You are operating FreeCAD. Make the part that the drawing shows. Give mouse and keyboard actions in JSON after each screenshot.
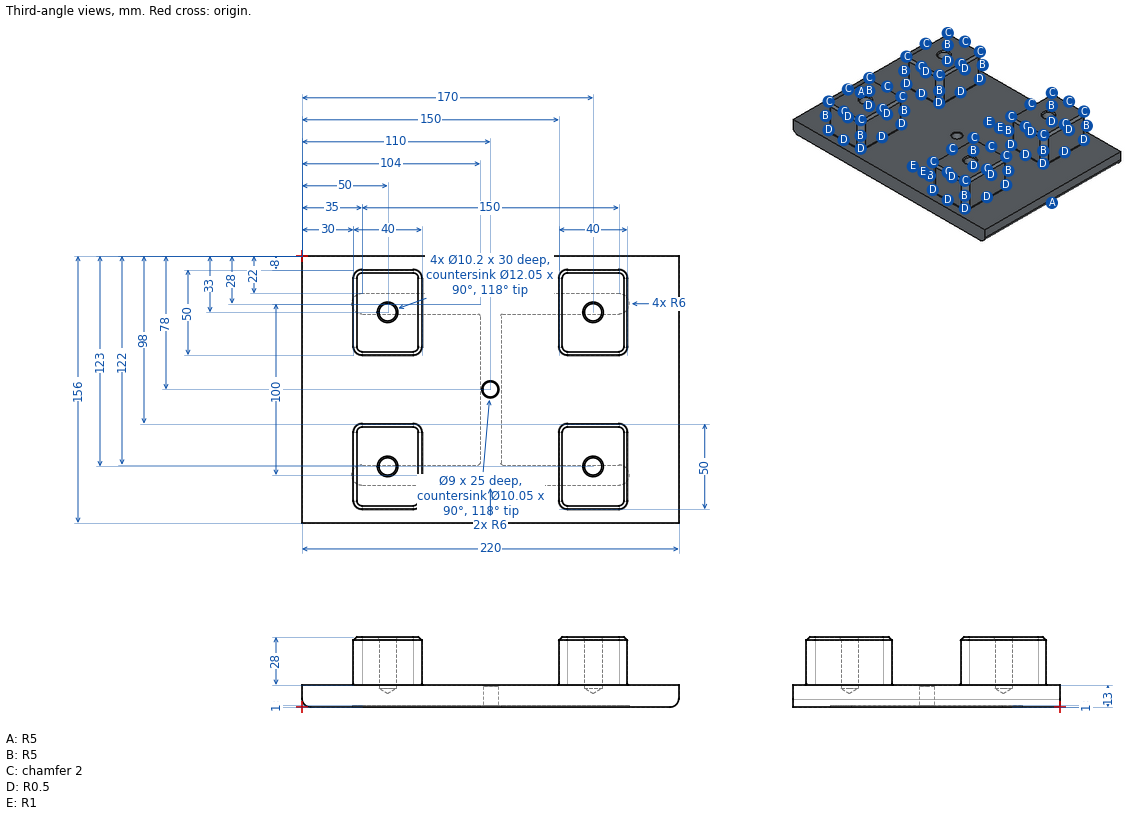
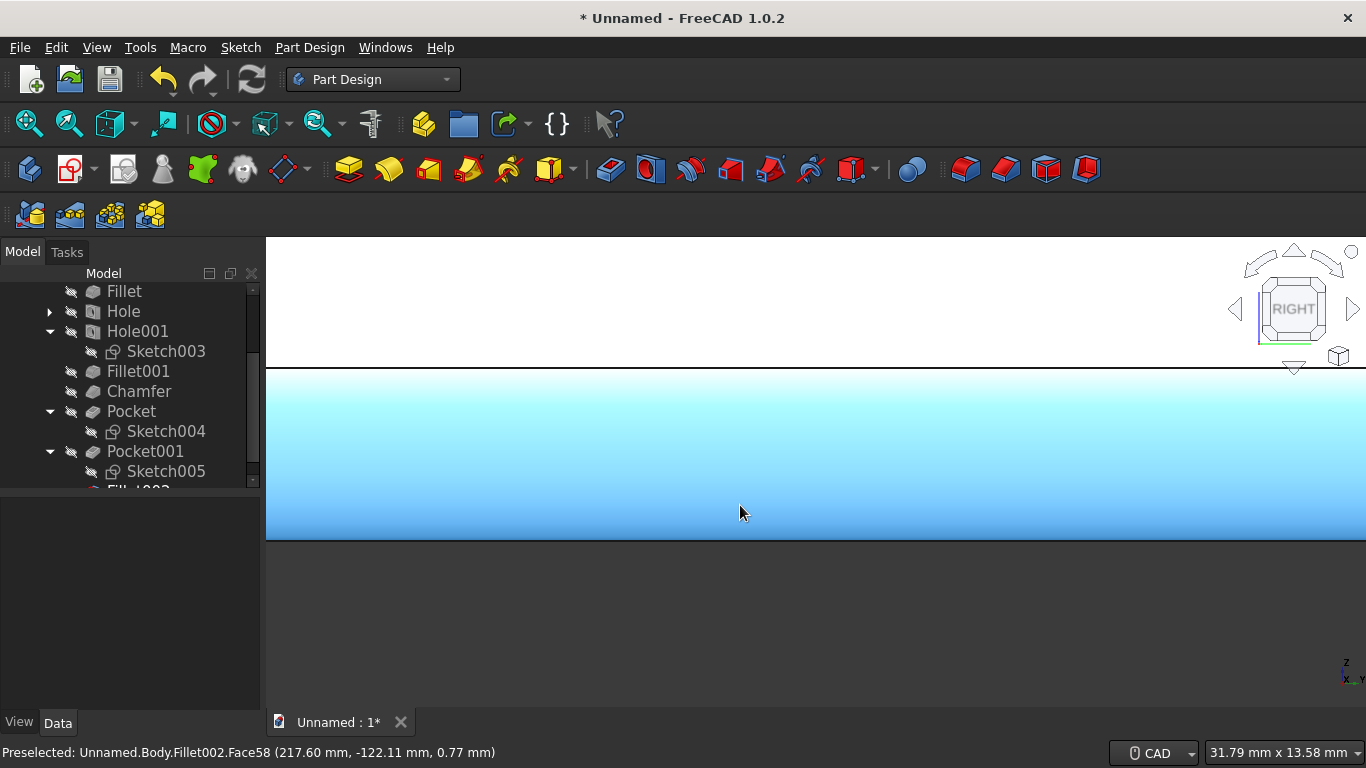
{"action": "key", "text": "v f"}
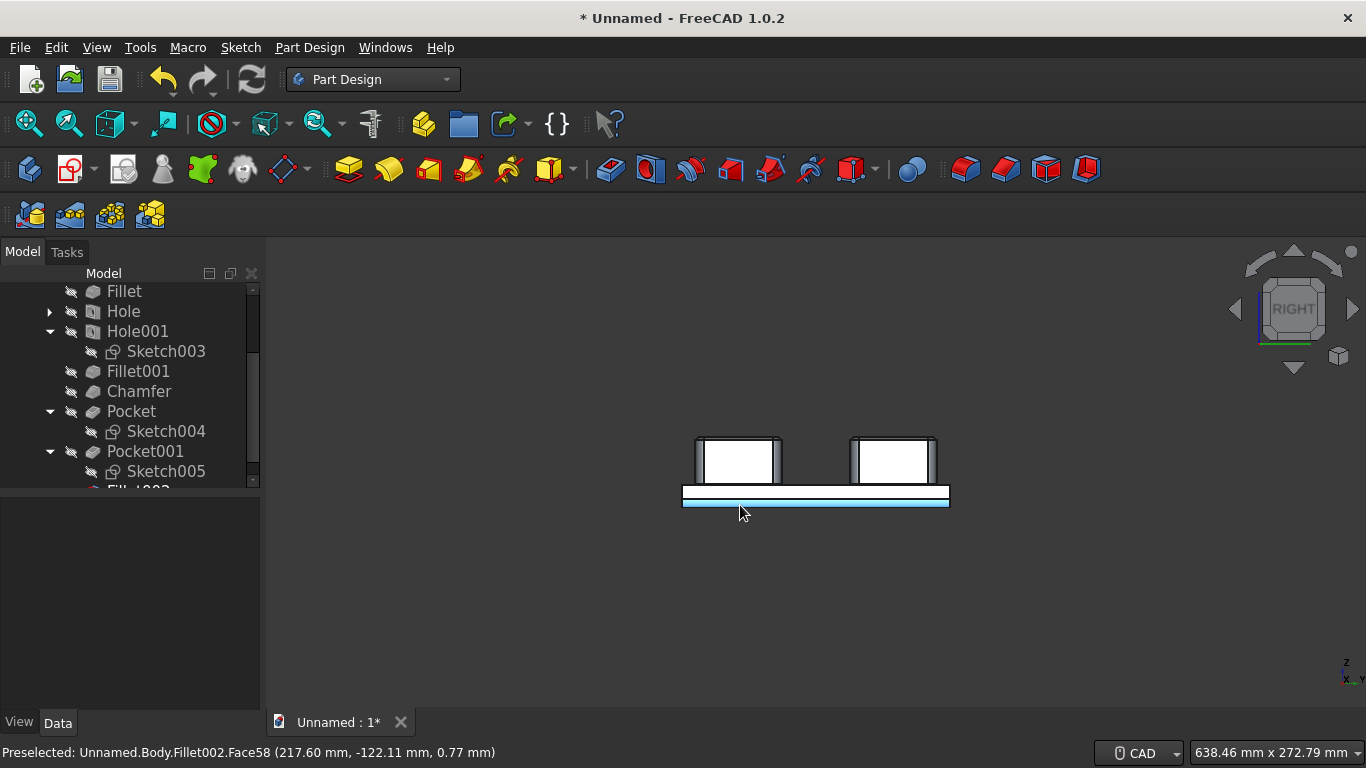
{"action": "key", "text": "5"}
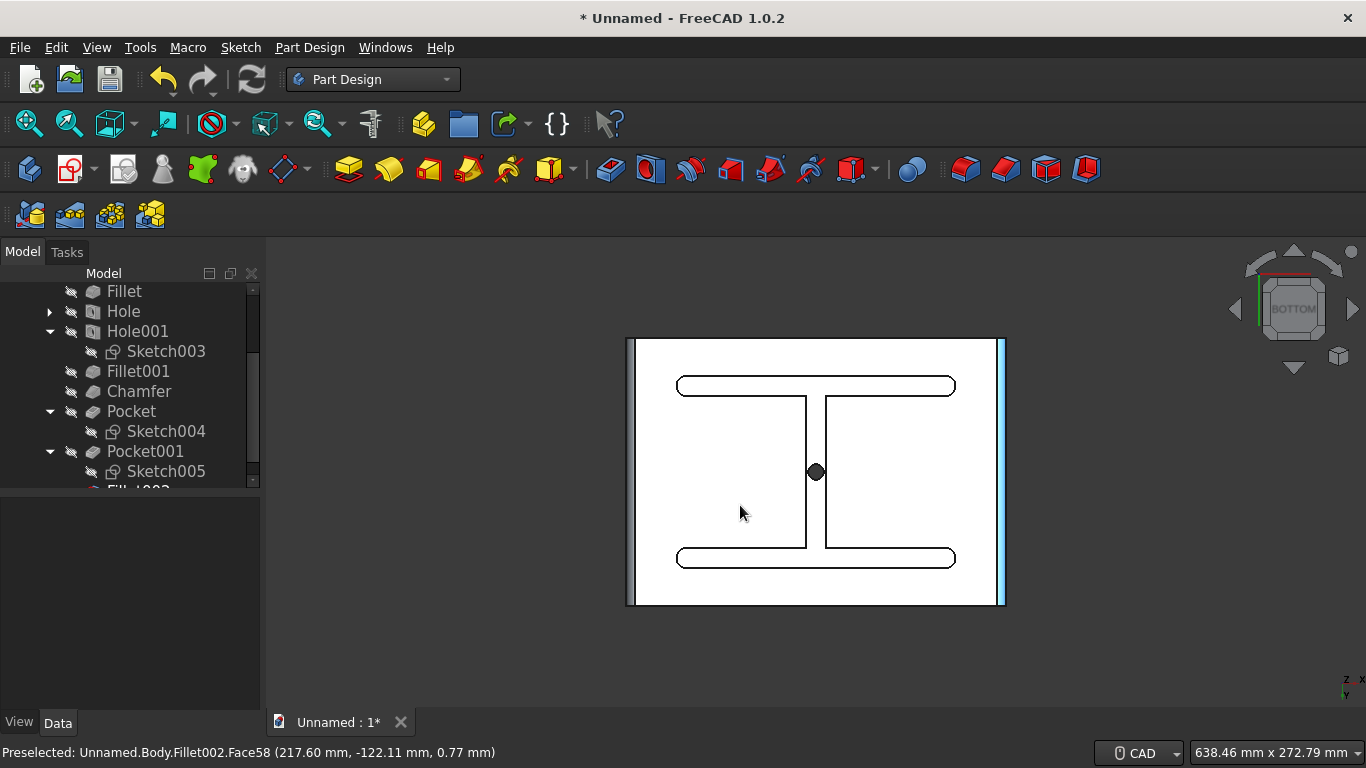
{"action": "scroll", "coordinate": [806, 395], "scroll_direction": "up", "scroll_amount": 15}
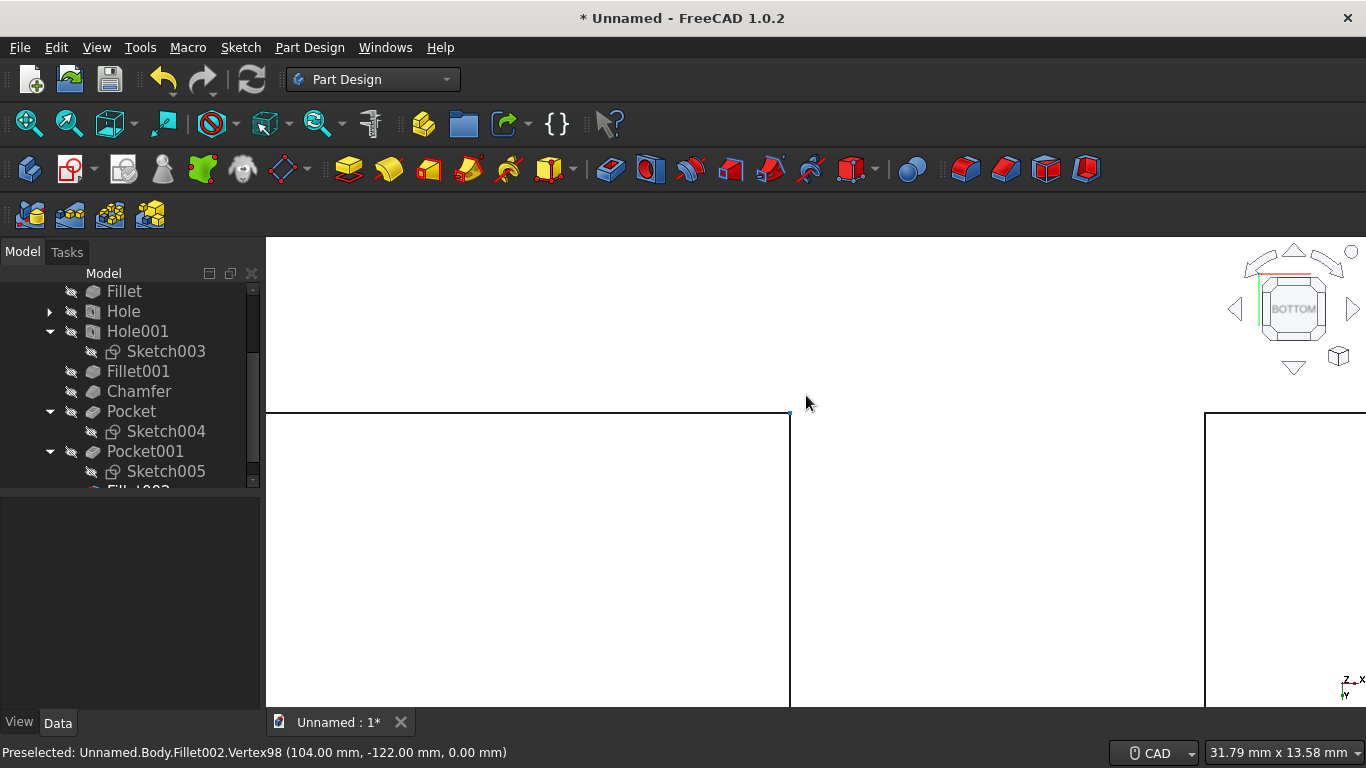
{"action": "key", "text": "v f"}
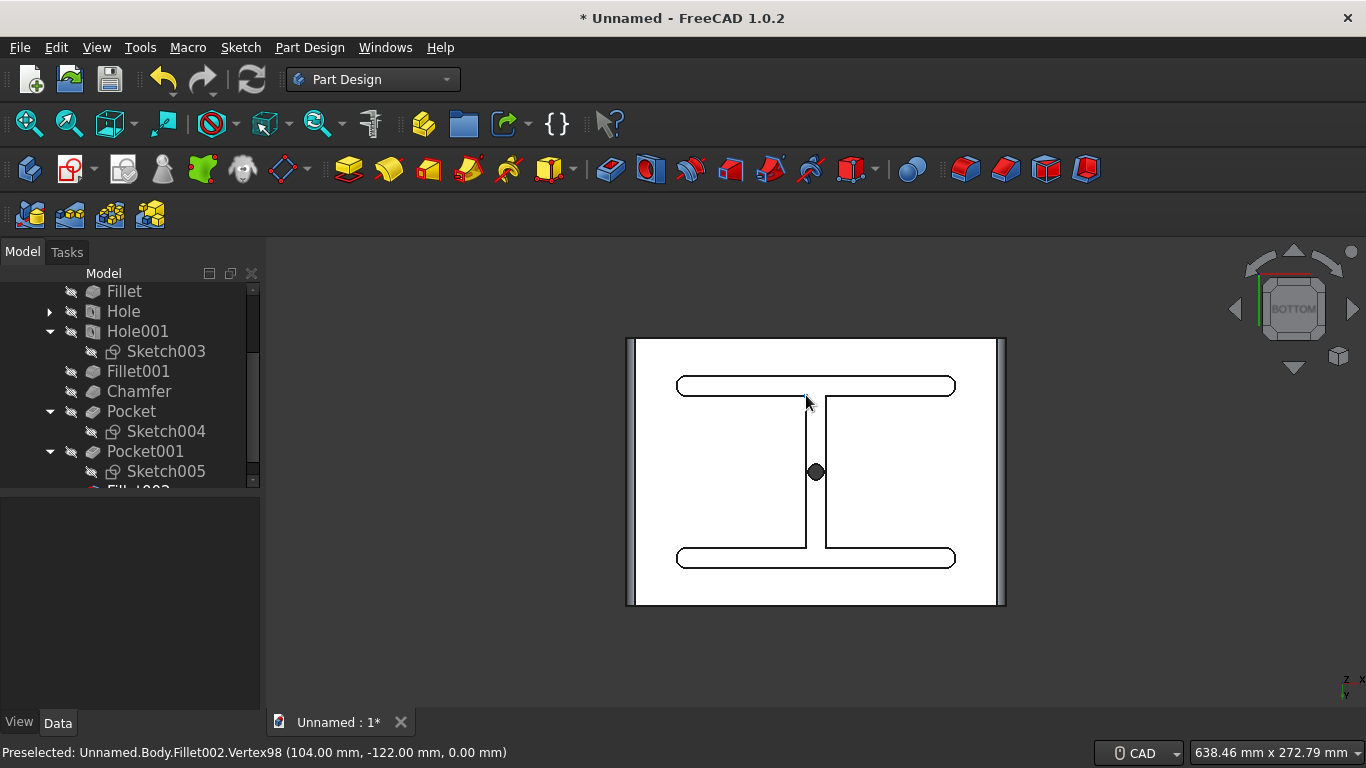
{"action": "key", "text": "4"}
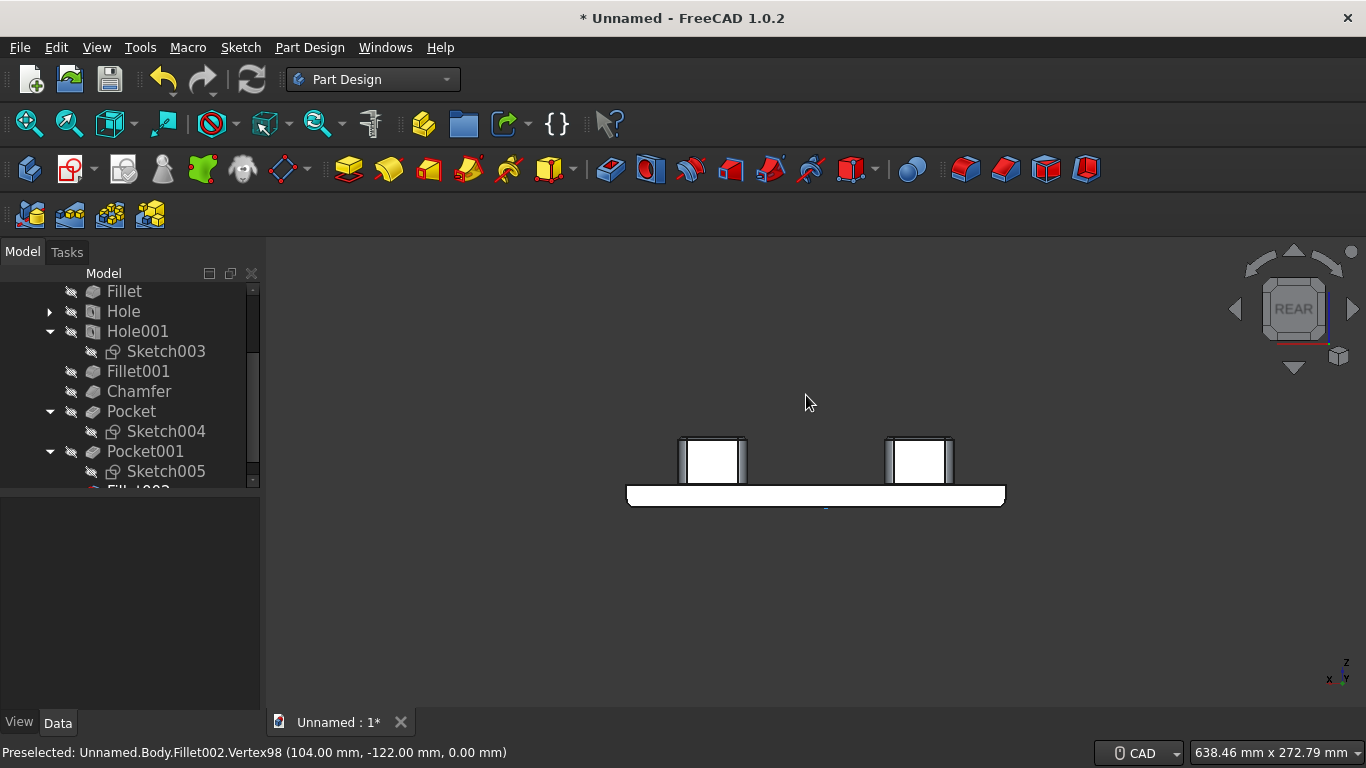
{"action": "key", "text": "v f"}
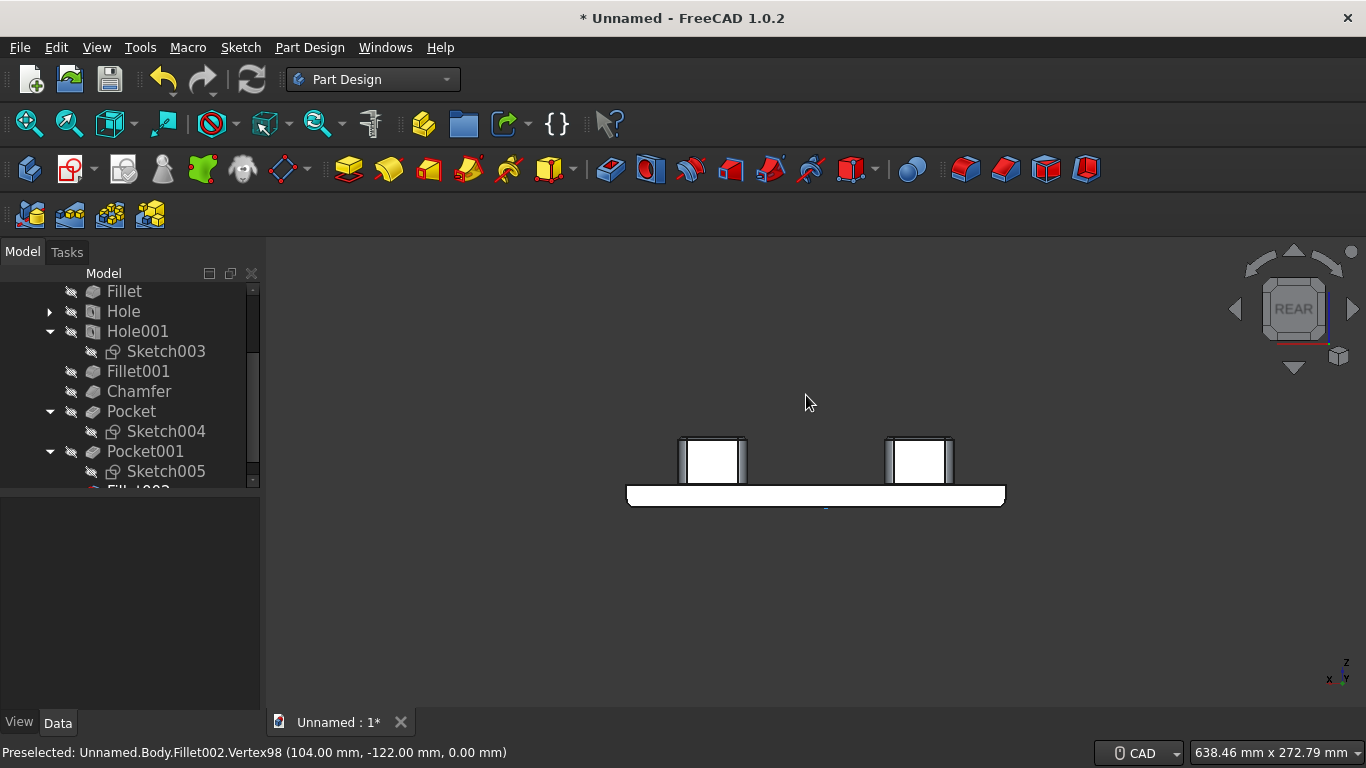
{"action": "scroll", "coordinate": [826, 505], "scroll_direction": "up", "scroll_amount": 15}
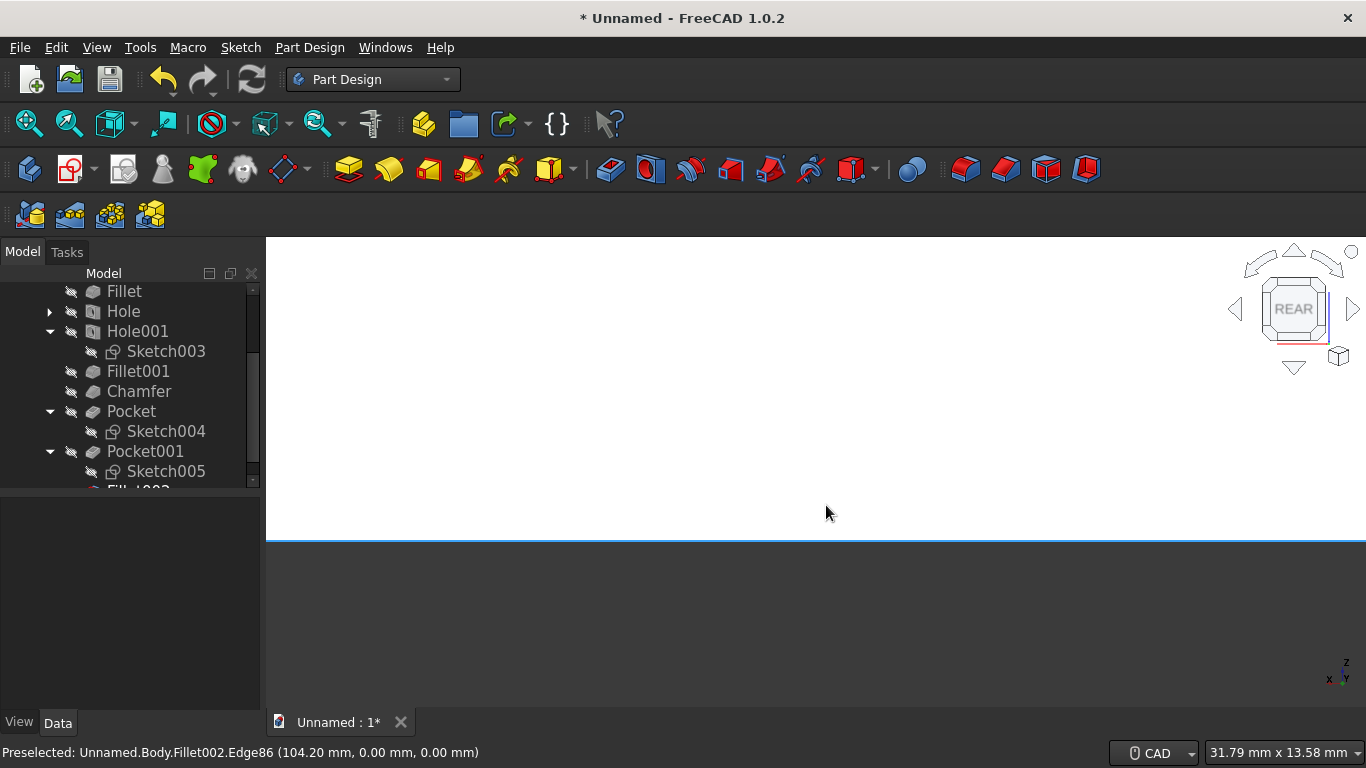
{"action": "left_click", "coordinate": [30, 124]}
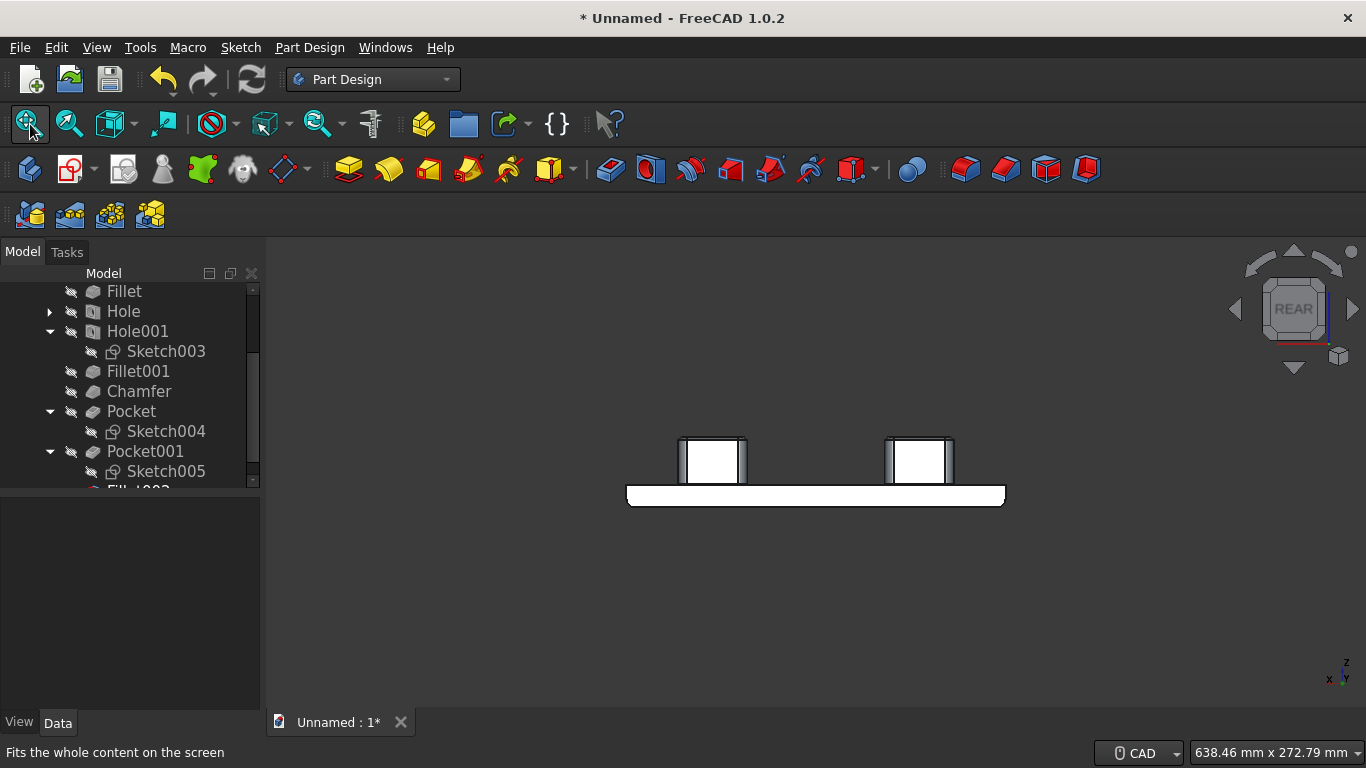
{"action": "key", "text": "6"}